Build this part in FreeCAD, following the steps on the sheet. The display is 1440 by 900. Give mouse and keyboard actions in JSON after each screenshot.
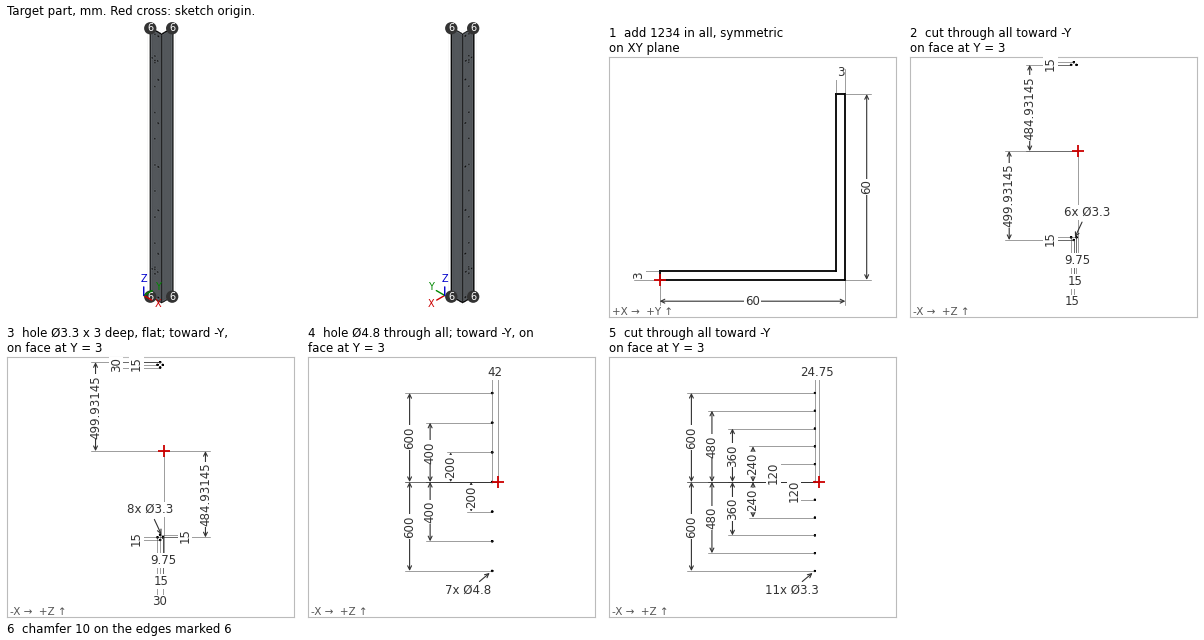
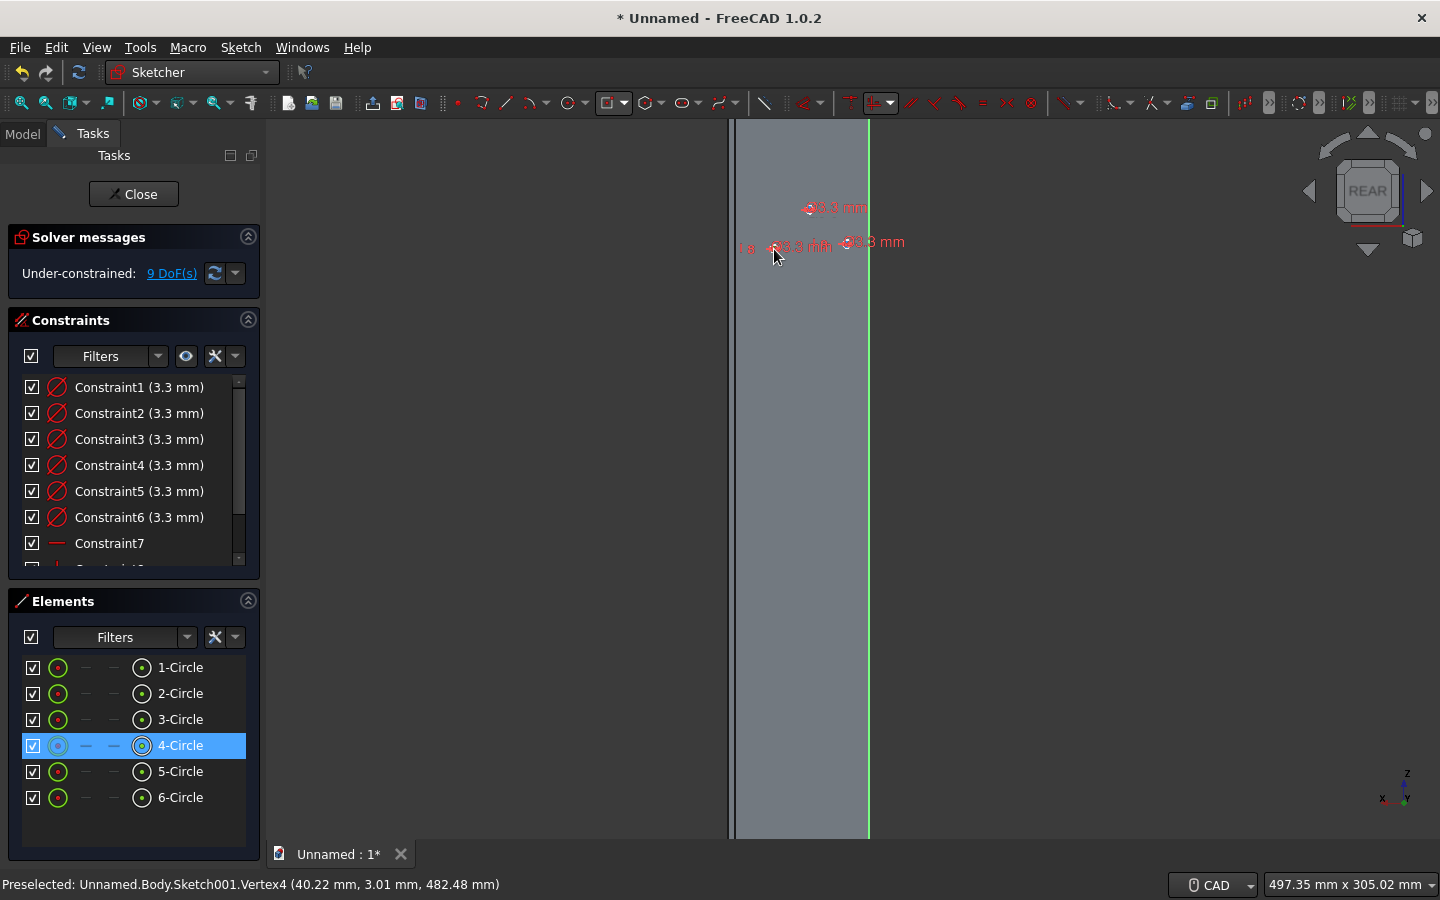
{"action": "scroll", "coordinate": [775, 249], "scroll_direction": "down", "scroll_amount": 8}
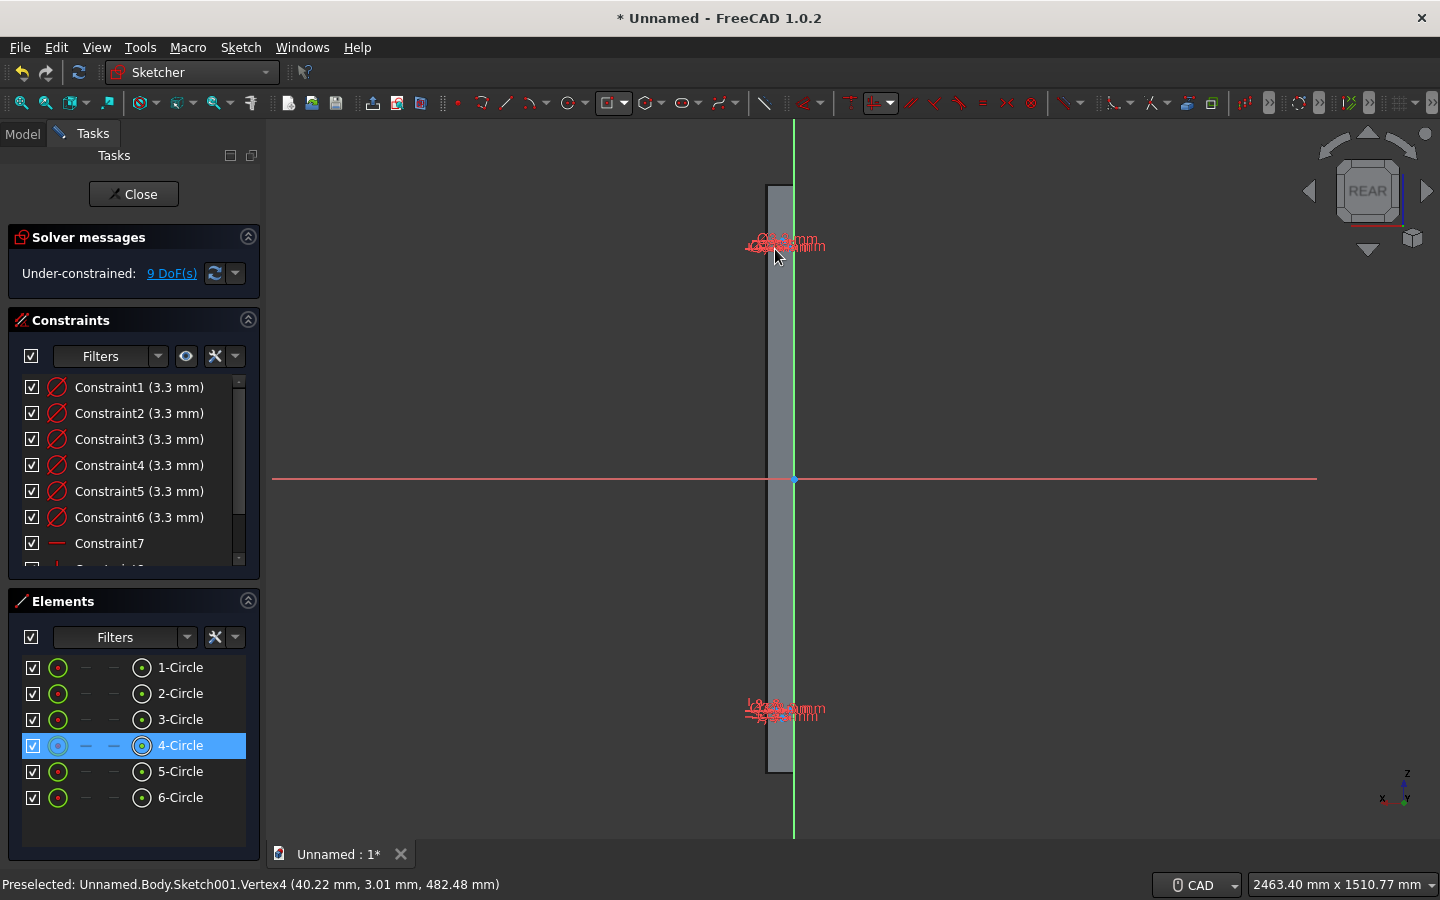
{"action": "left_click", "coordinate": [790, 248]}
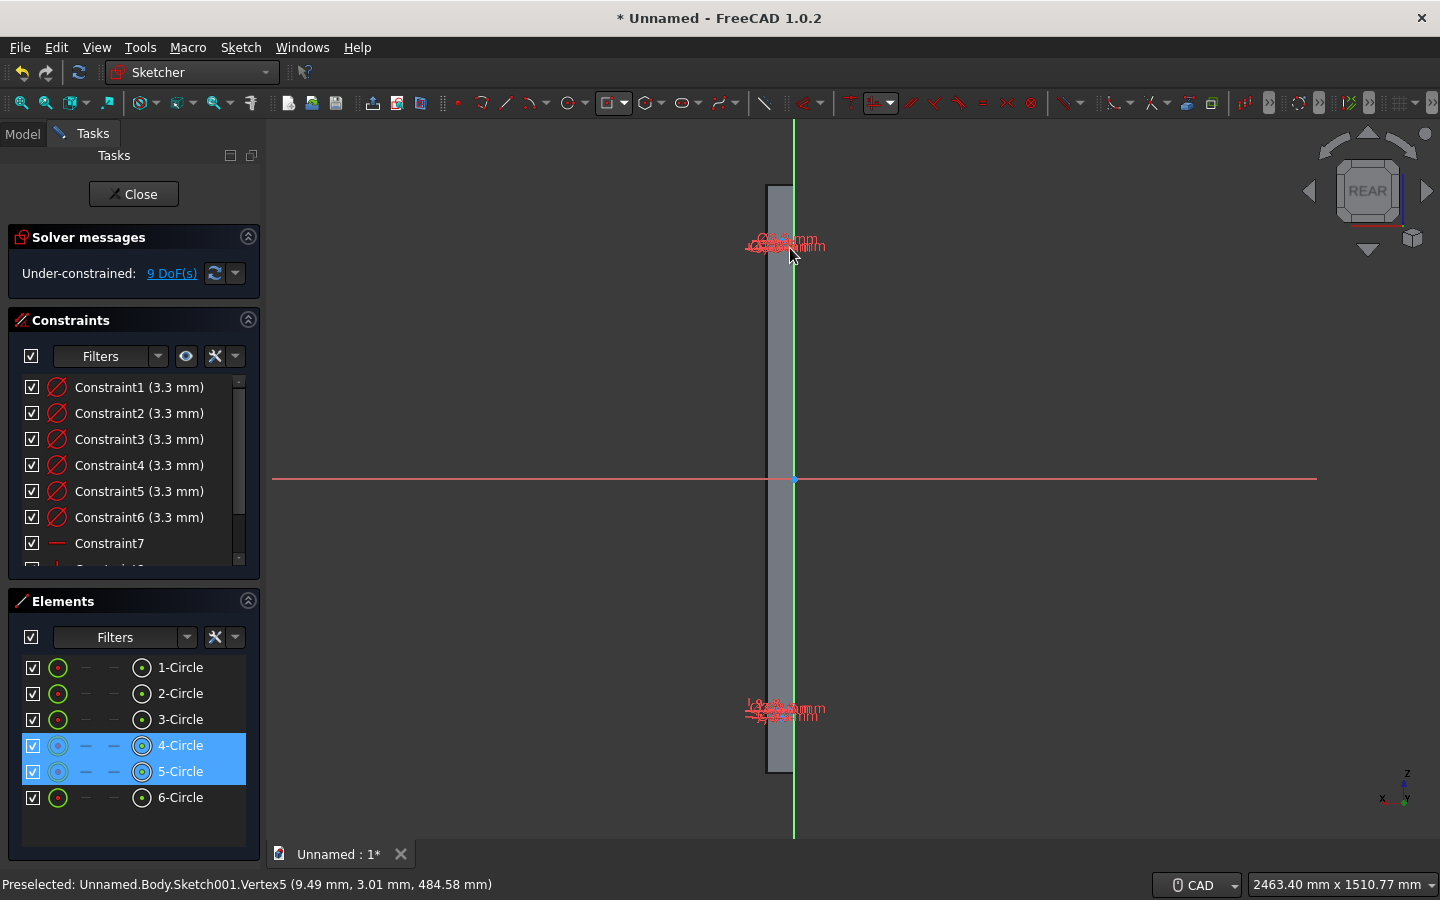
{"action": "left_click", "coordinate": [892, 104]}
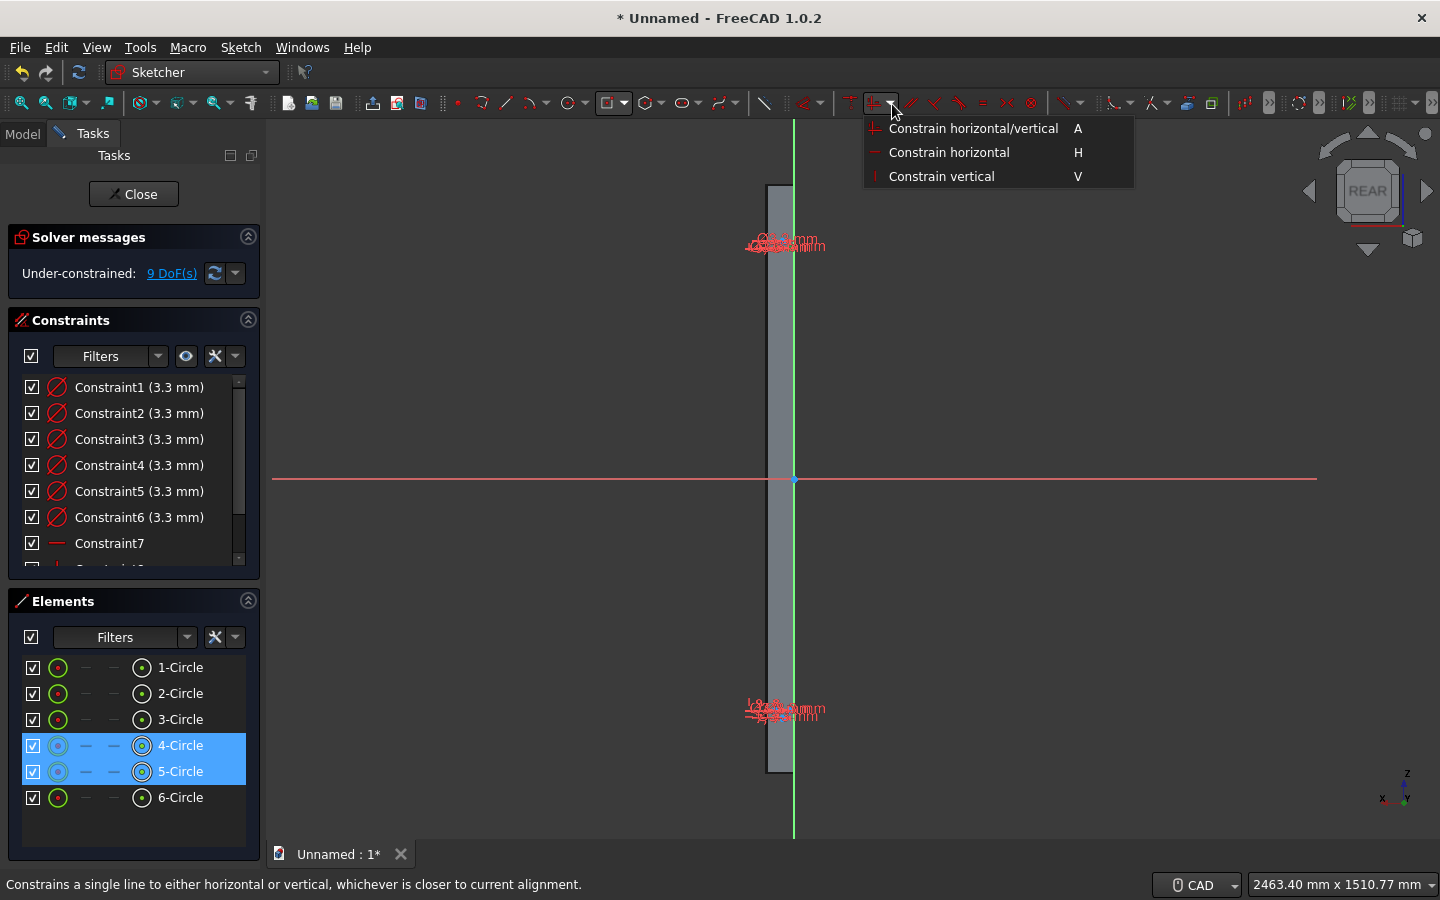
{"action": "left_click", "coordinate": [999, 152]}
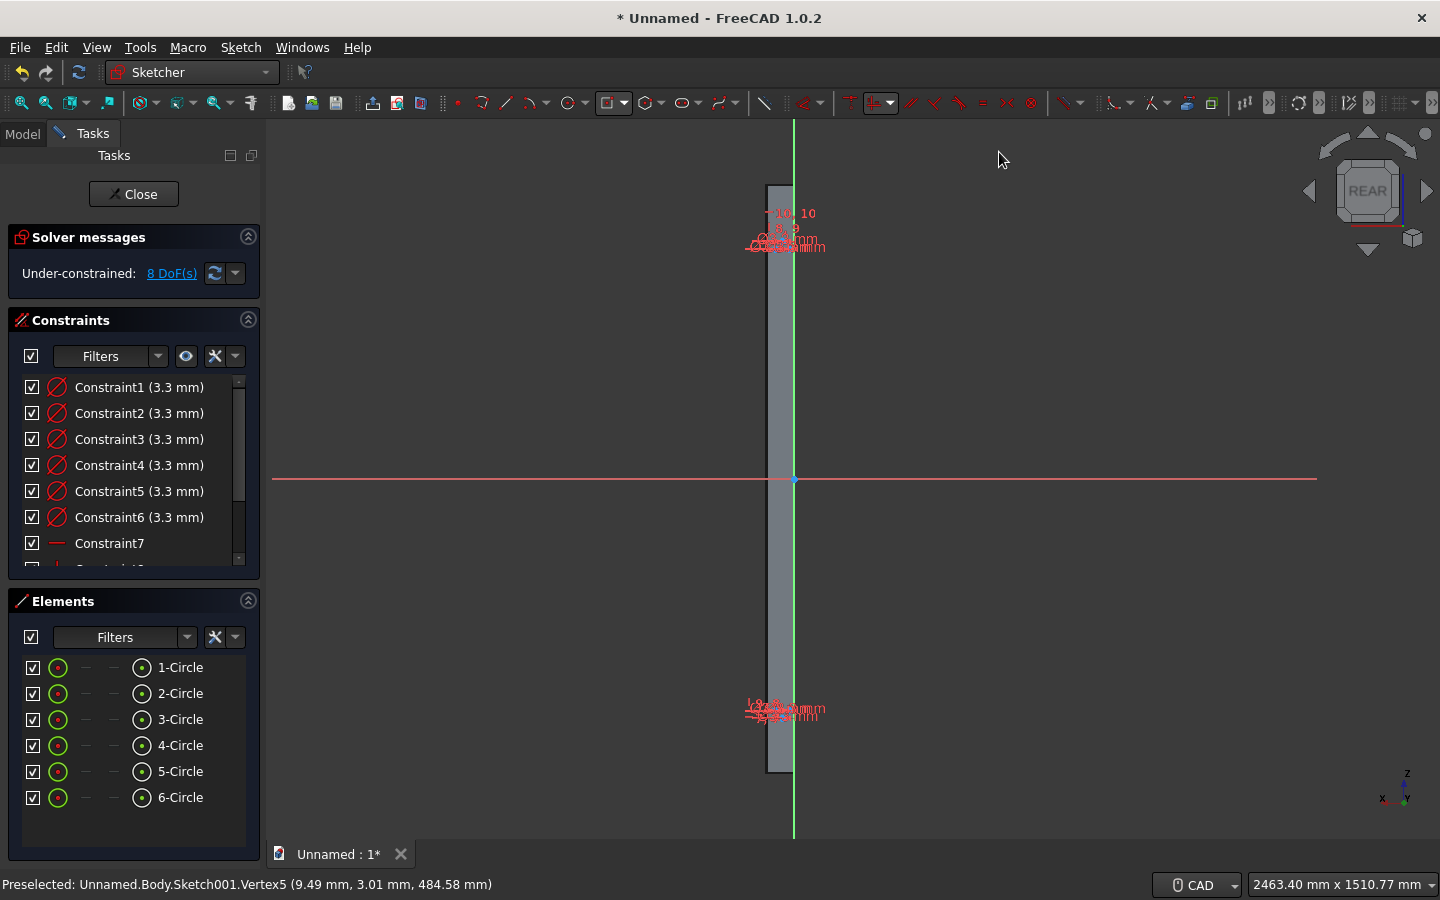
{"action": "left_click", "coordinate": [782, 718]}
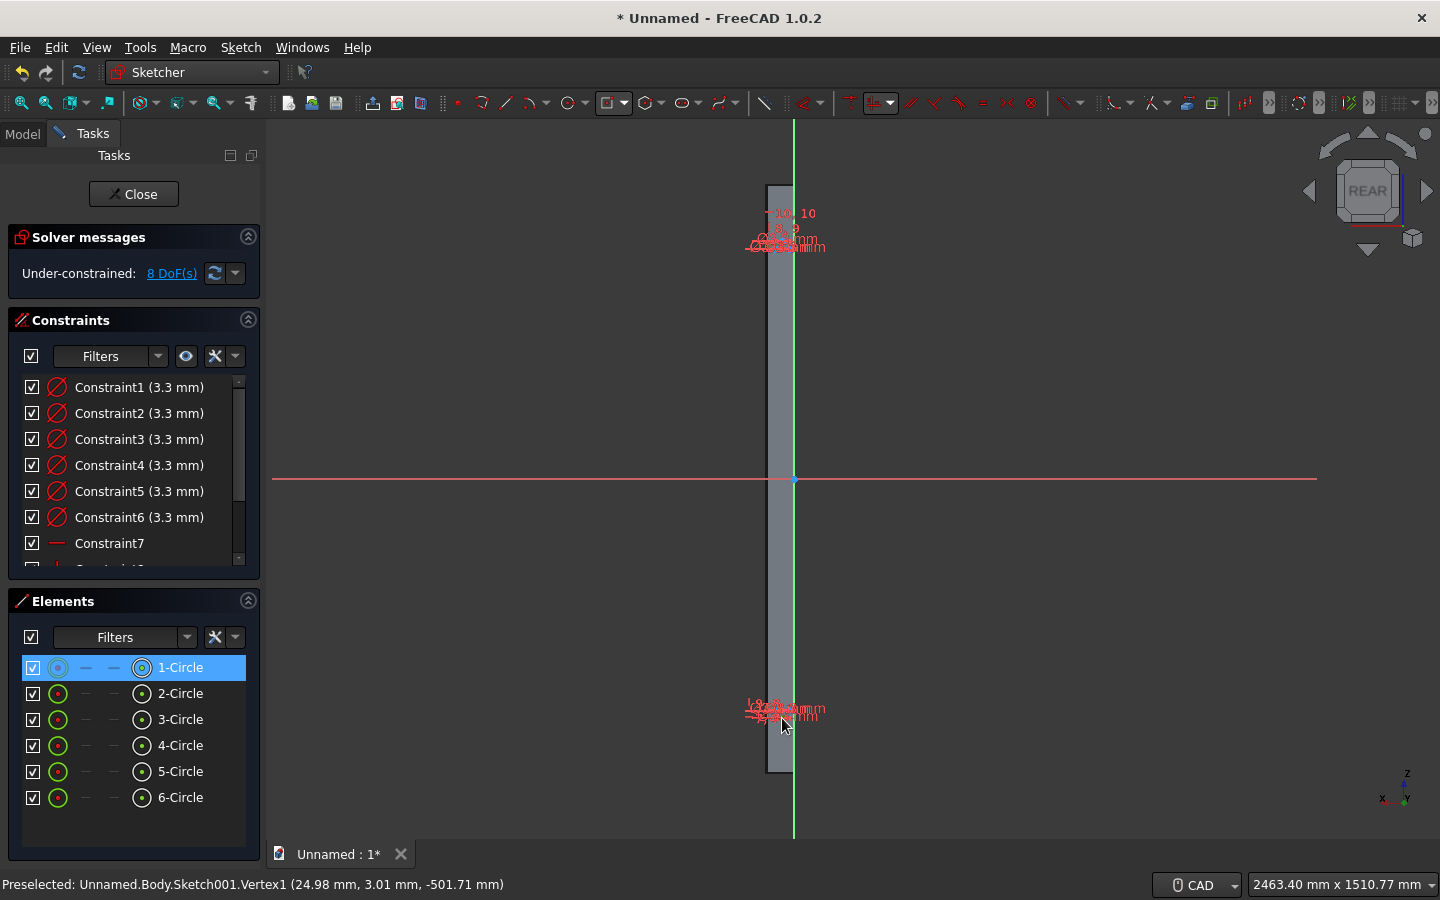
{"action": "left_click", "coordinate": [782, 241]}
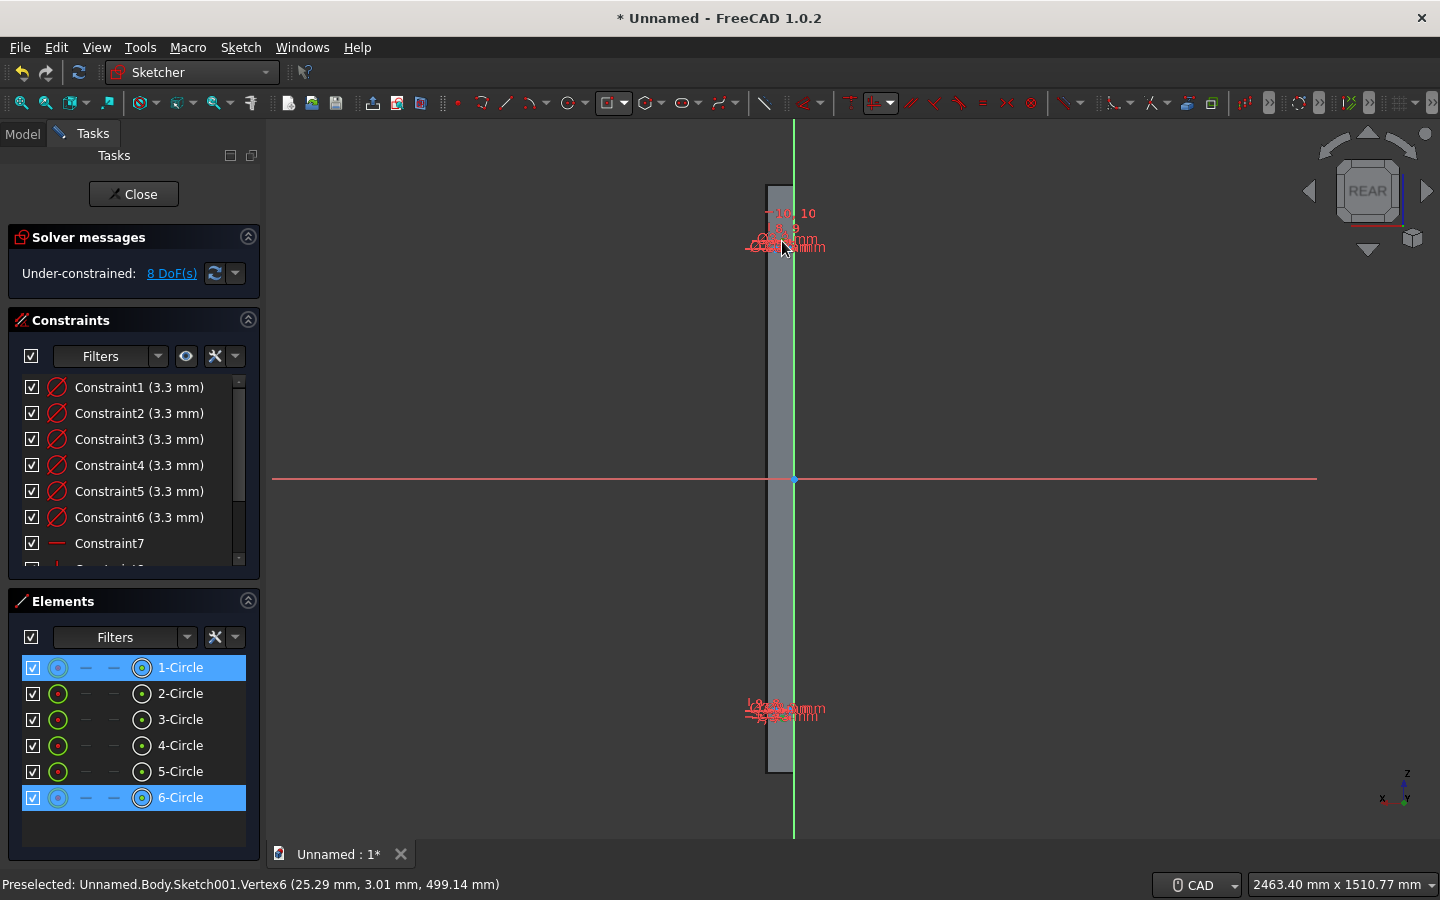
{"action": "key", "text": "v"}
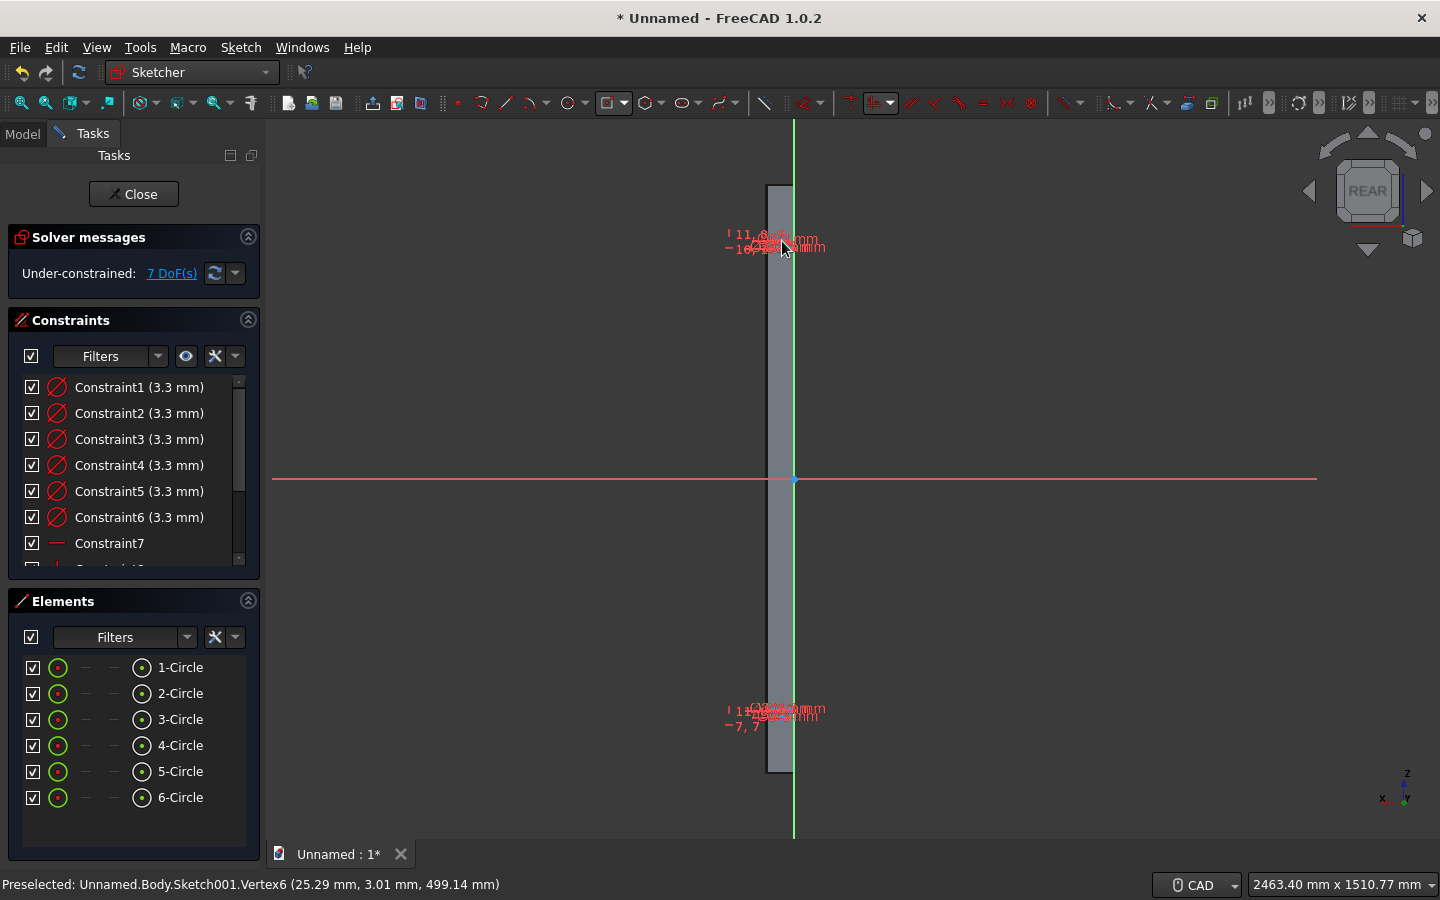
{"action": "left_click", "coordinate": [804, 104]}